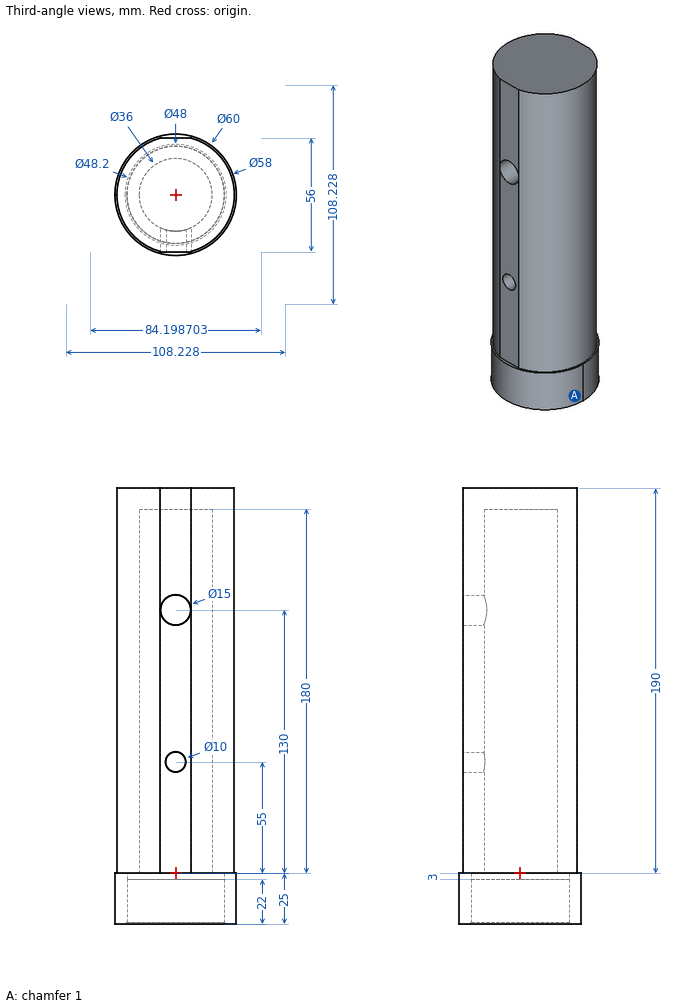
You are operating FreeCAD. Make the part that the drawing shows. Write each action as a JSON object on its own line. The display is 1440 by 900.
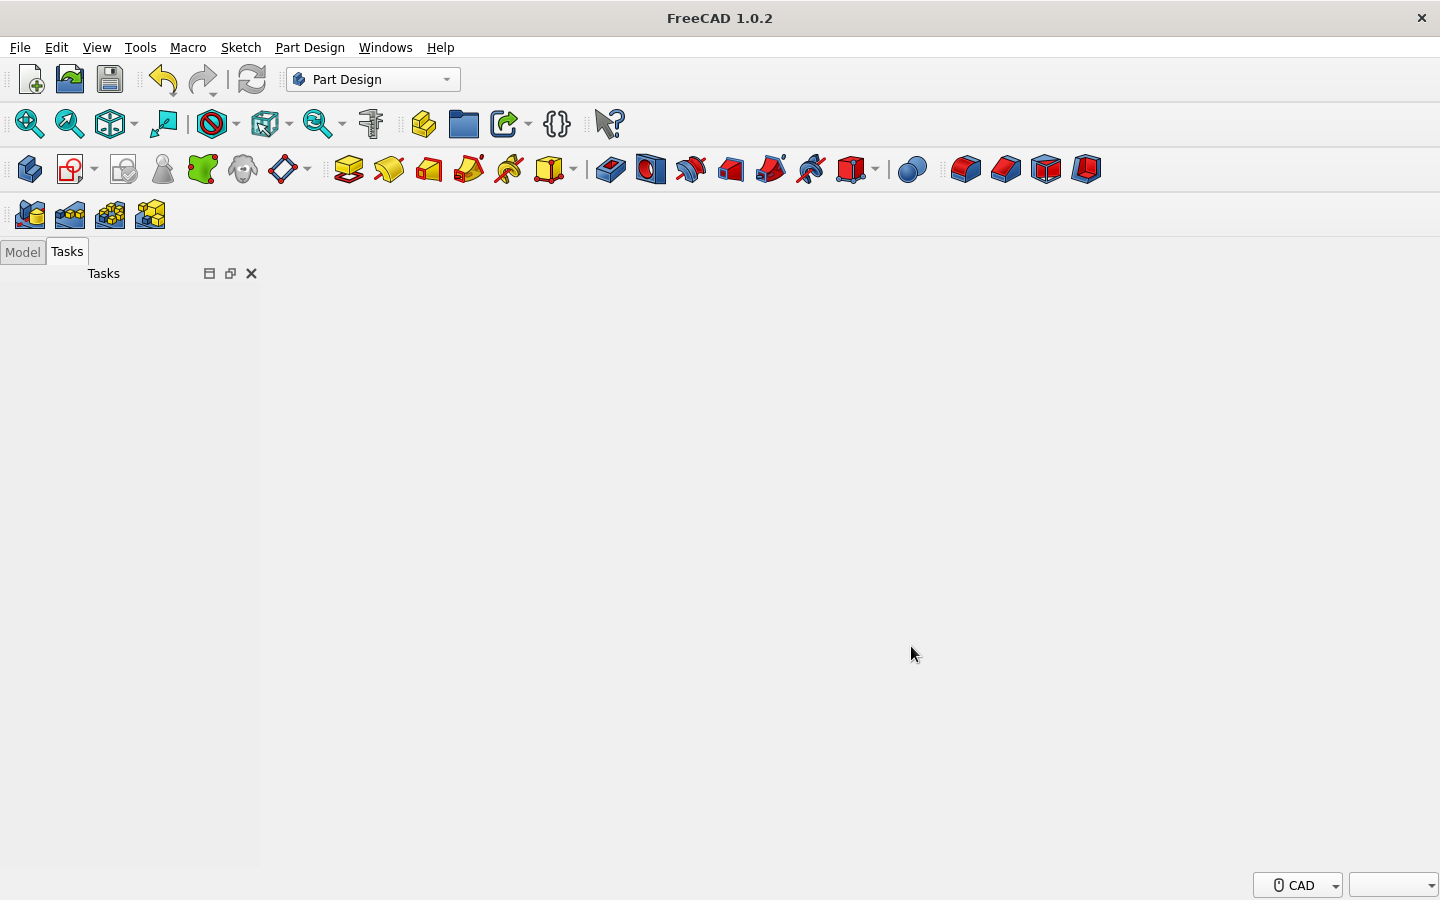
{"action": "left_click", "coordinate": [30, 80]}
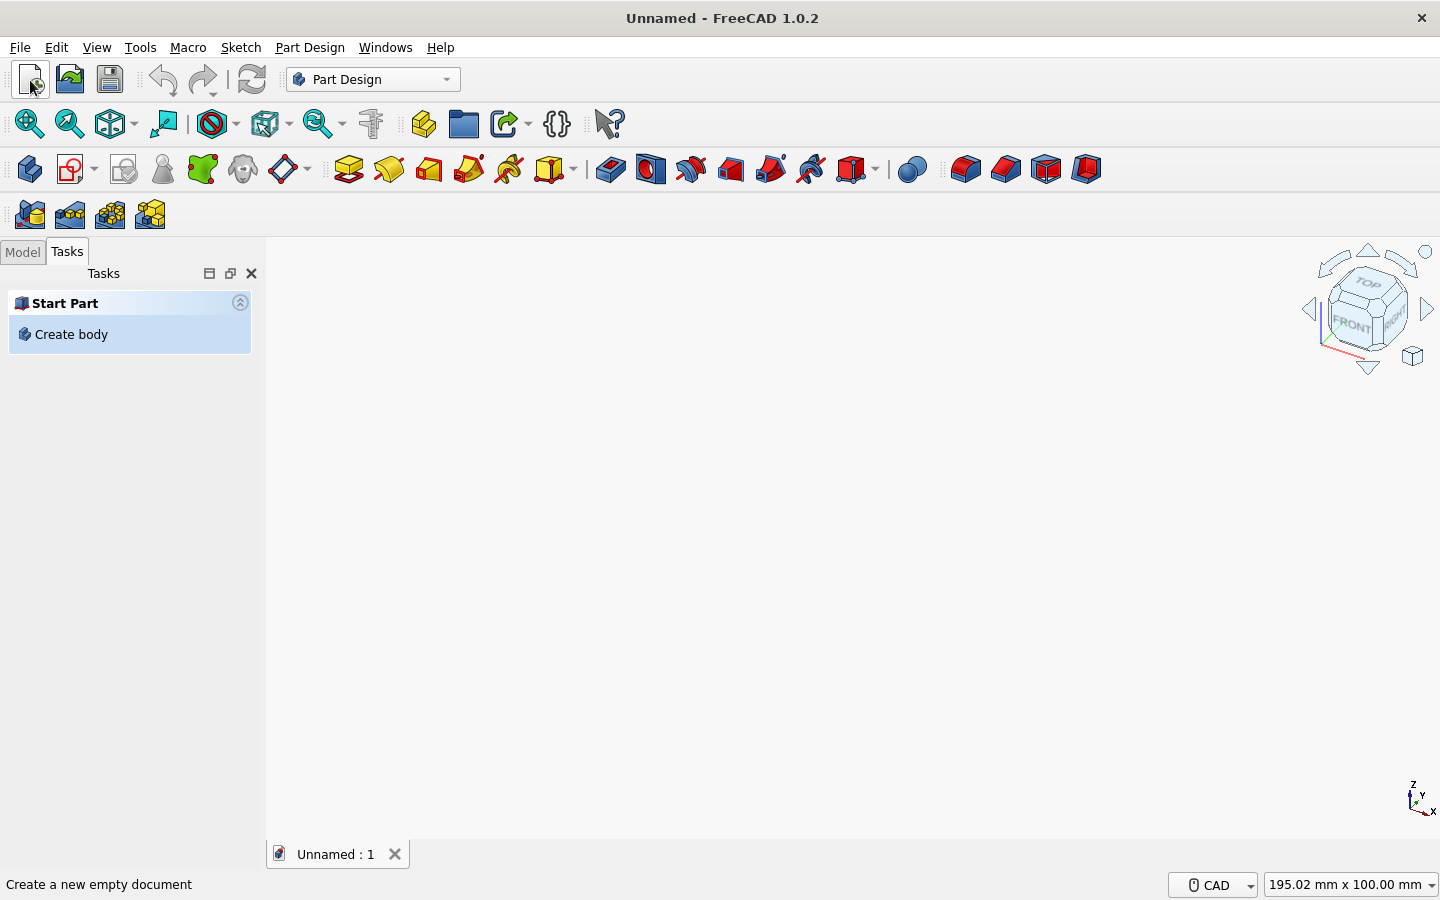
{"action": "left_click", "coordinate": [70, 170]}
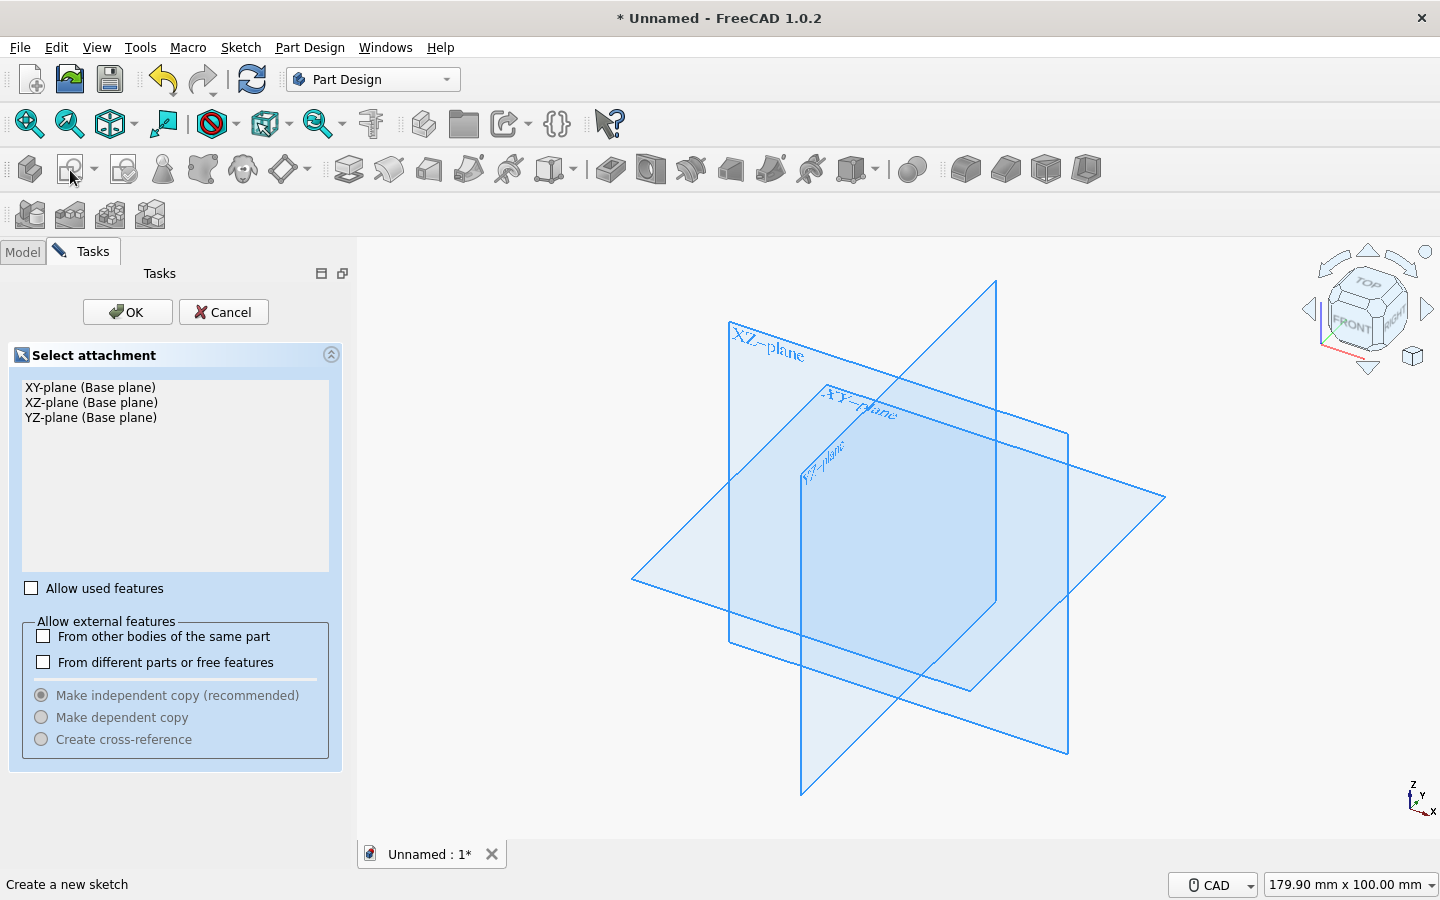
{"action": "left_click", "coordinate": [82, 388]}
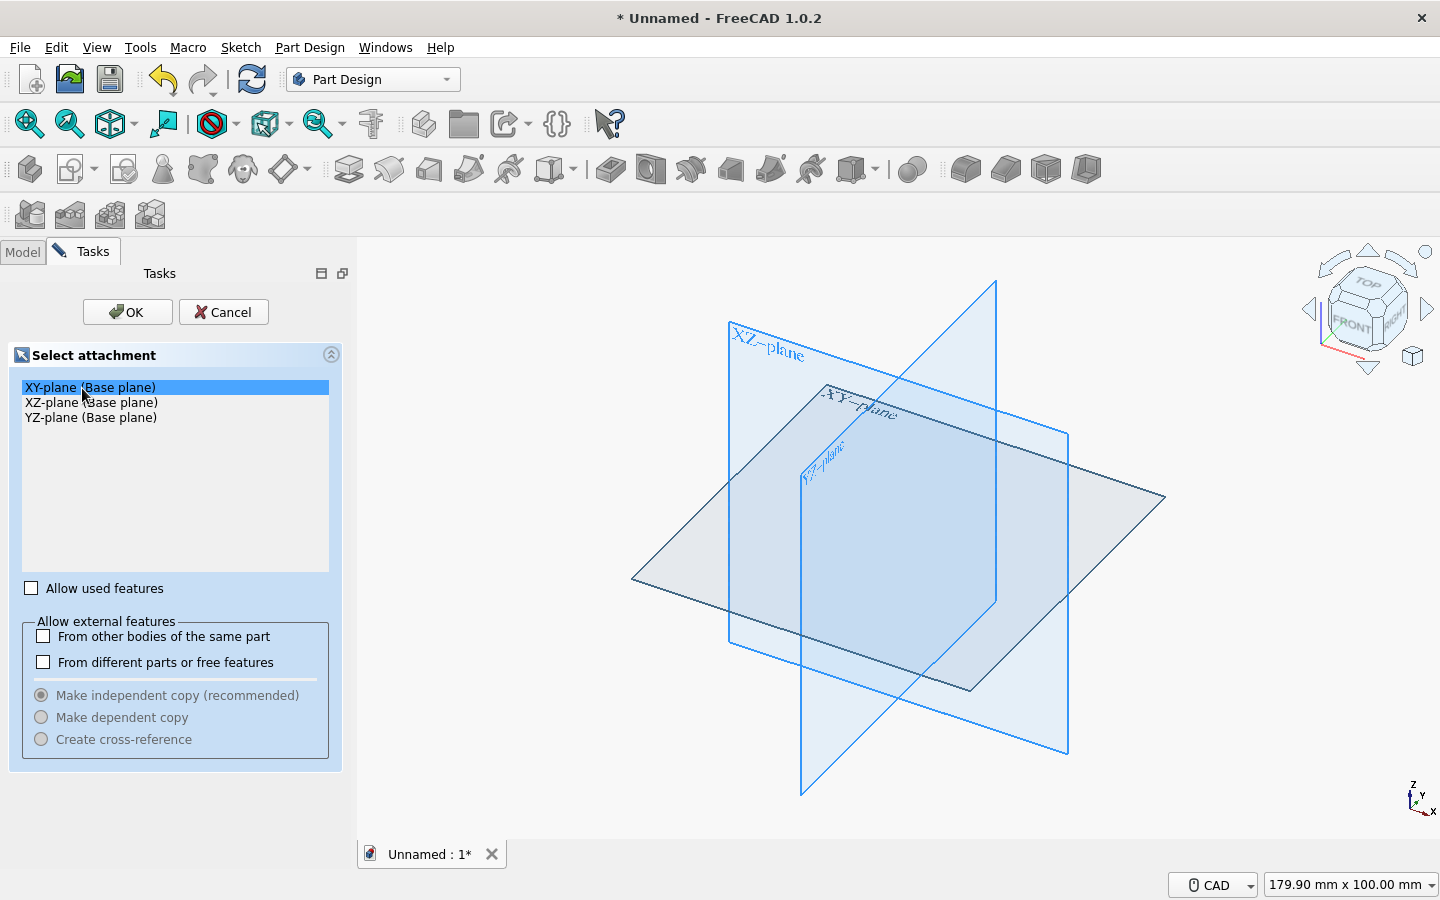
{"action": "left_click", "coordinate": [128, 312]}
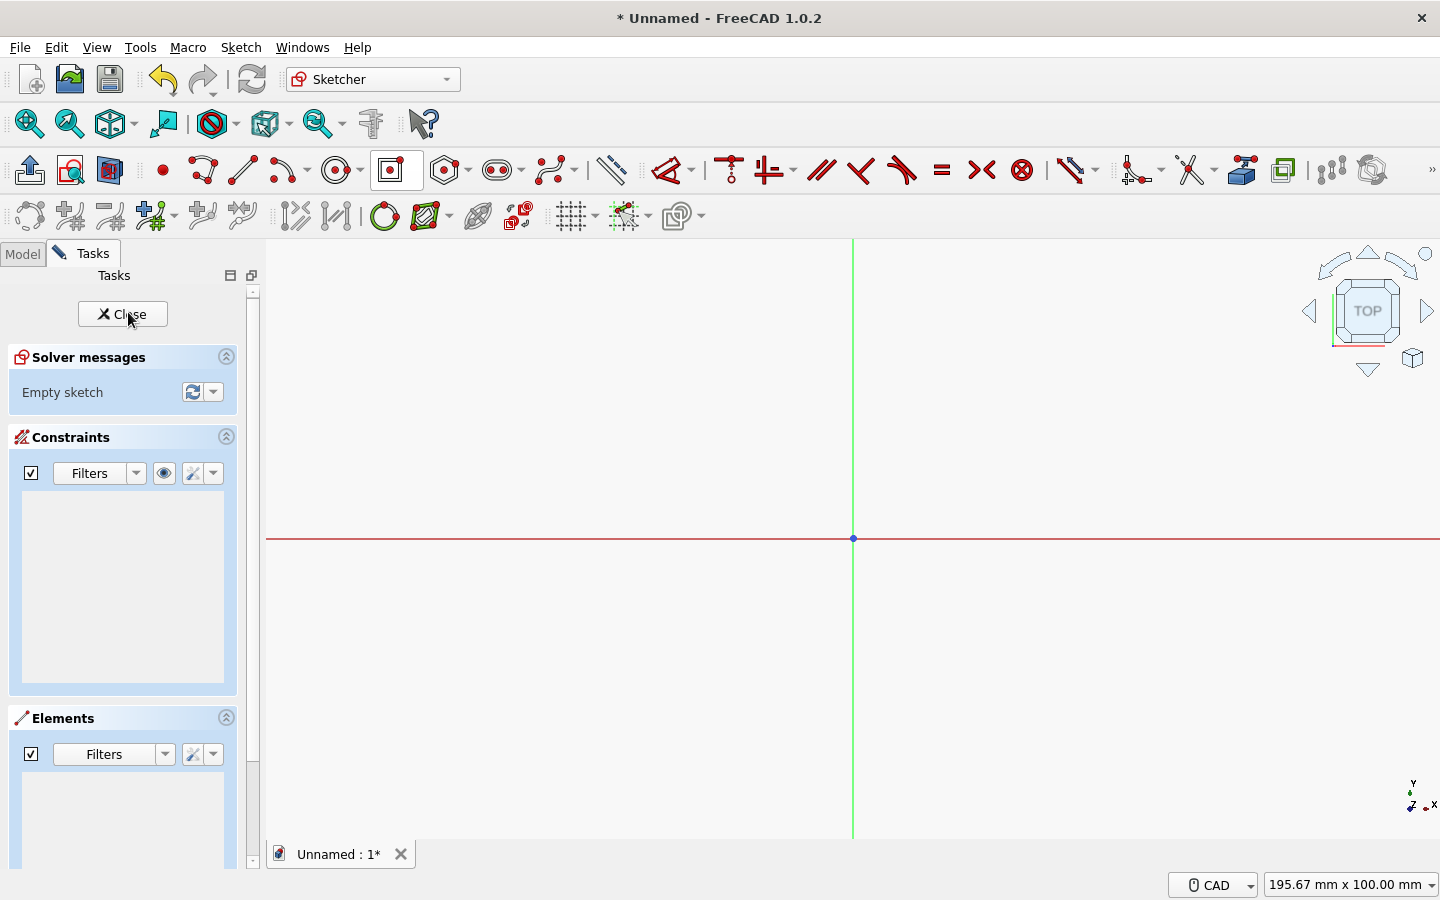
{"action": "left_click", "coordinate": [336, 170]}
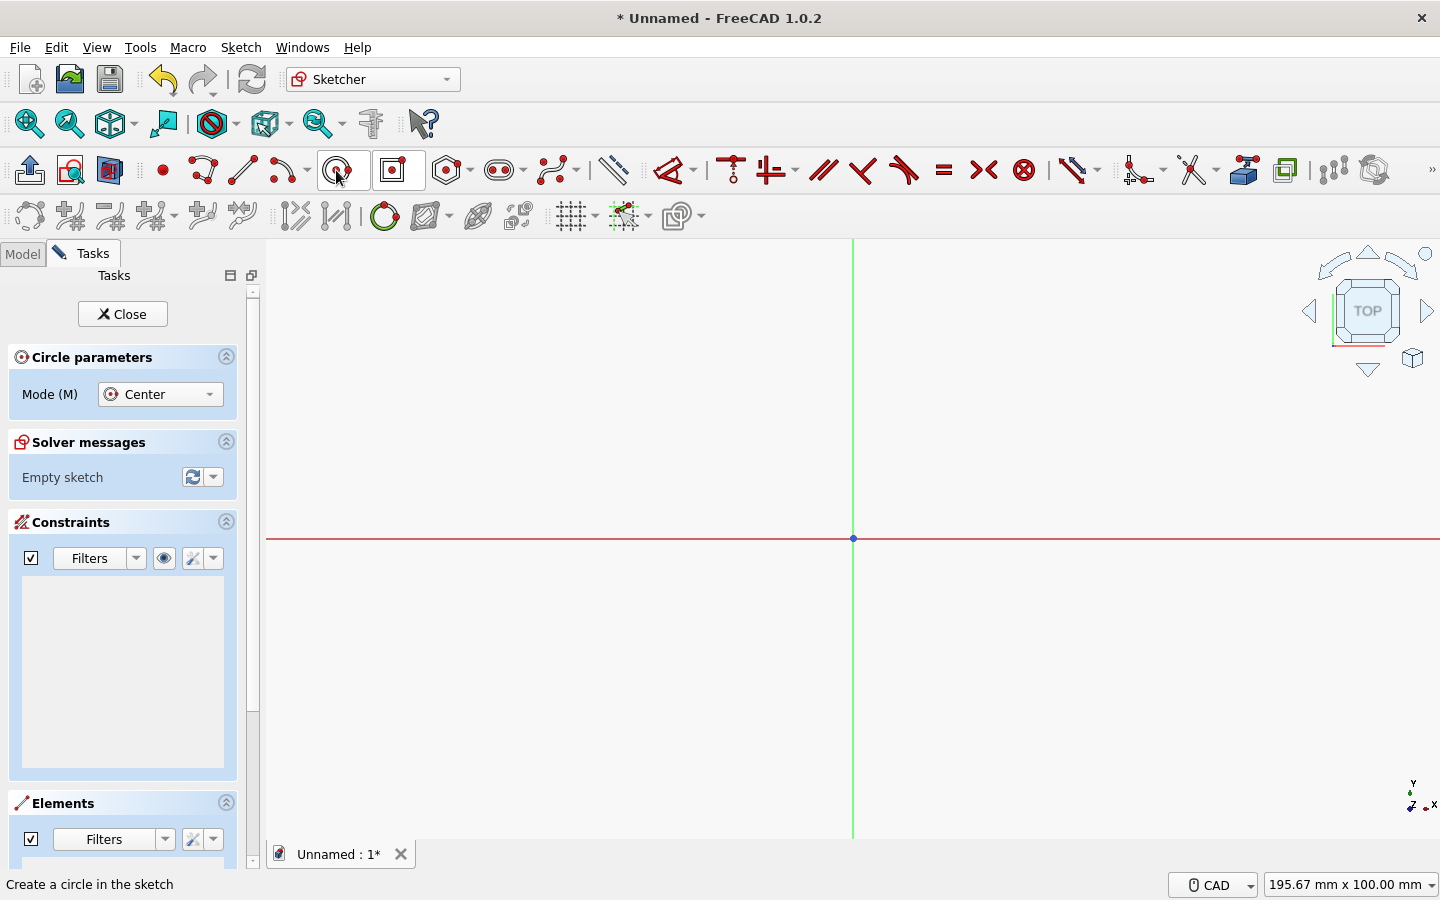
{"action": "left_click", "coordinate": [853, 539]}
{"action": "left_click", "coordinate": [976, 416]}
{"action": "key", "text": "Escape"}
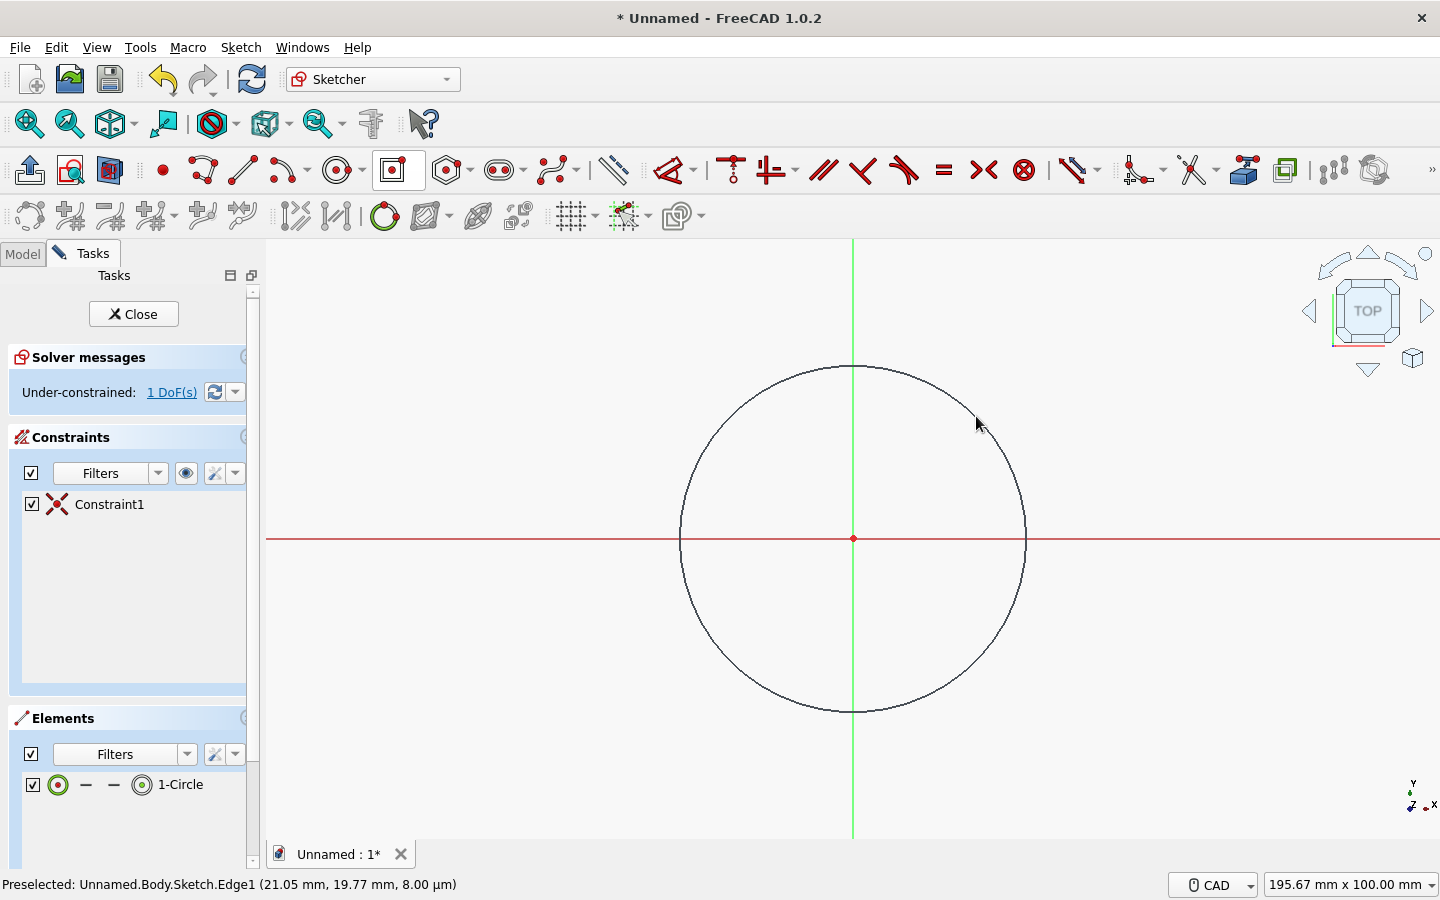
{"action": "left_click", "coordinate": [975, 416]}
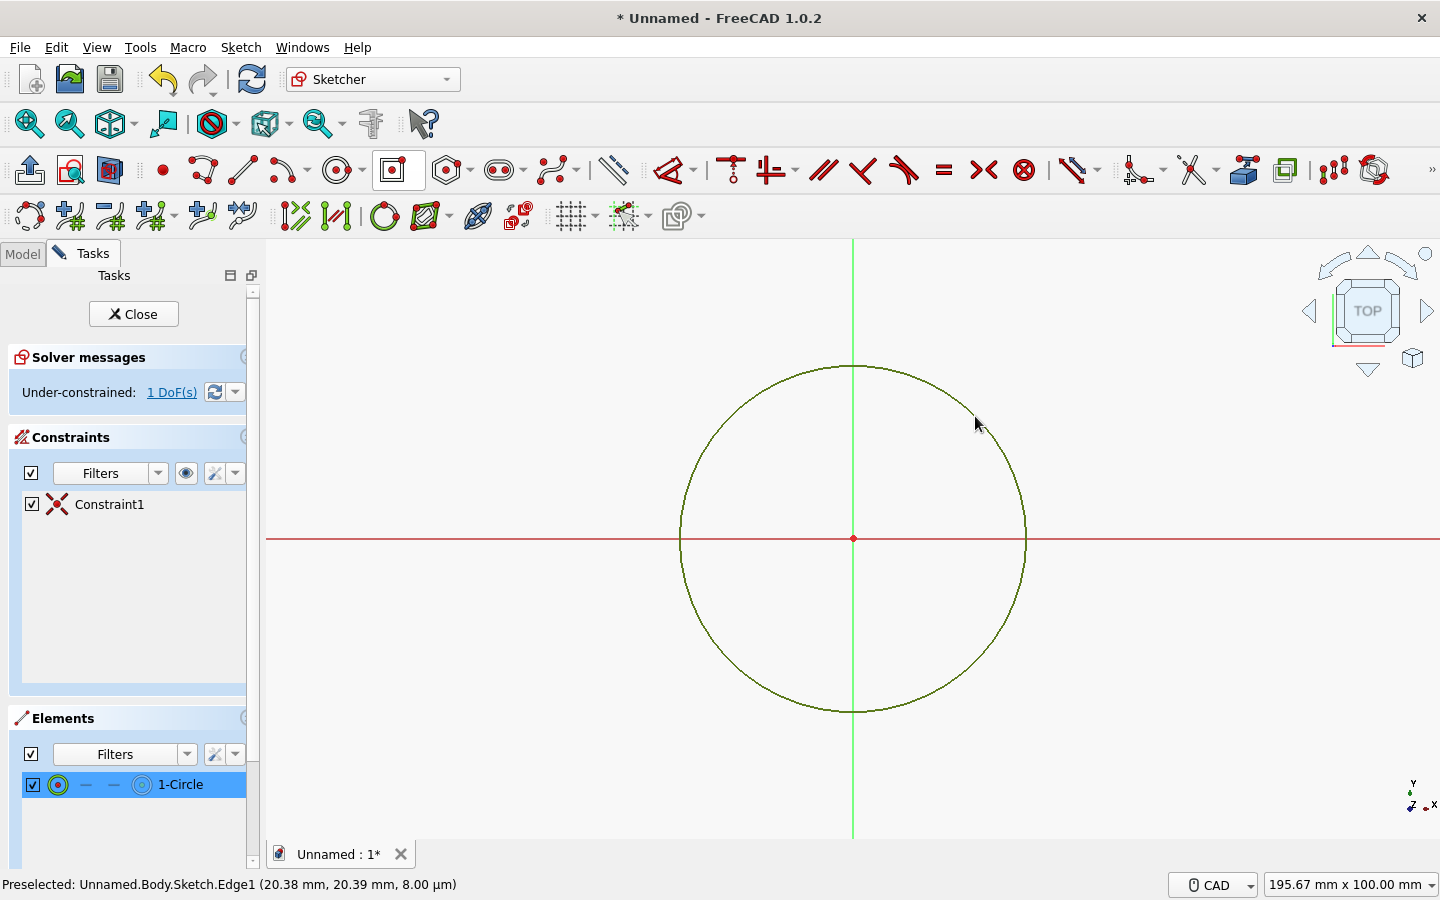
{"action": "key", "text": "k o"}